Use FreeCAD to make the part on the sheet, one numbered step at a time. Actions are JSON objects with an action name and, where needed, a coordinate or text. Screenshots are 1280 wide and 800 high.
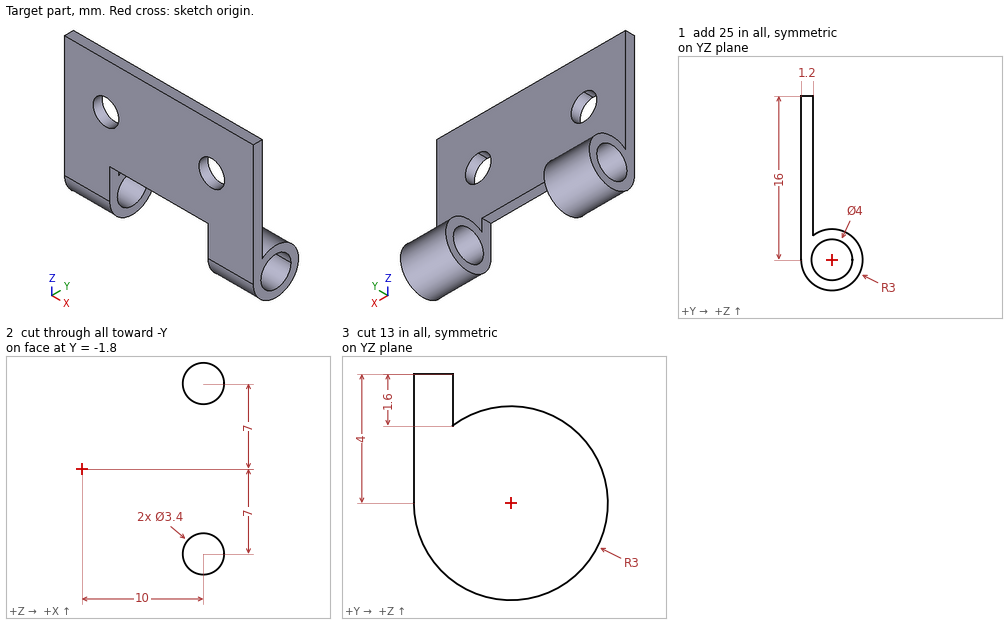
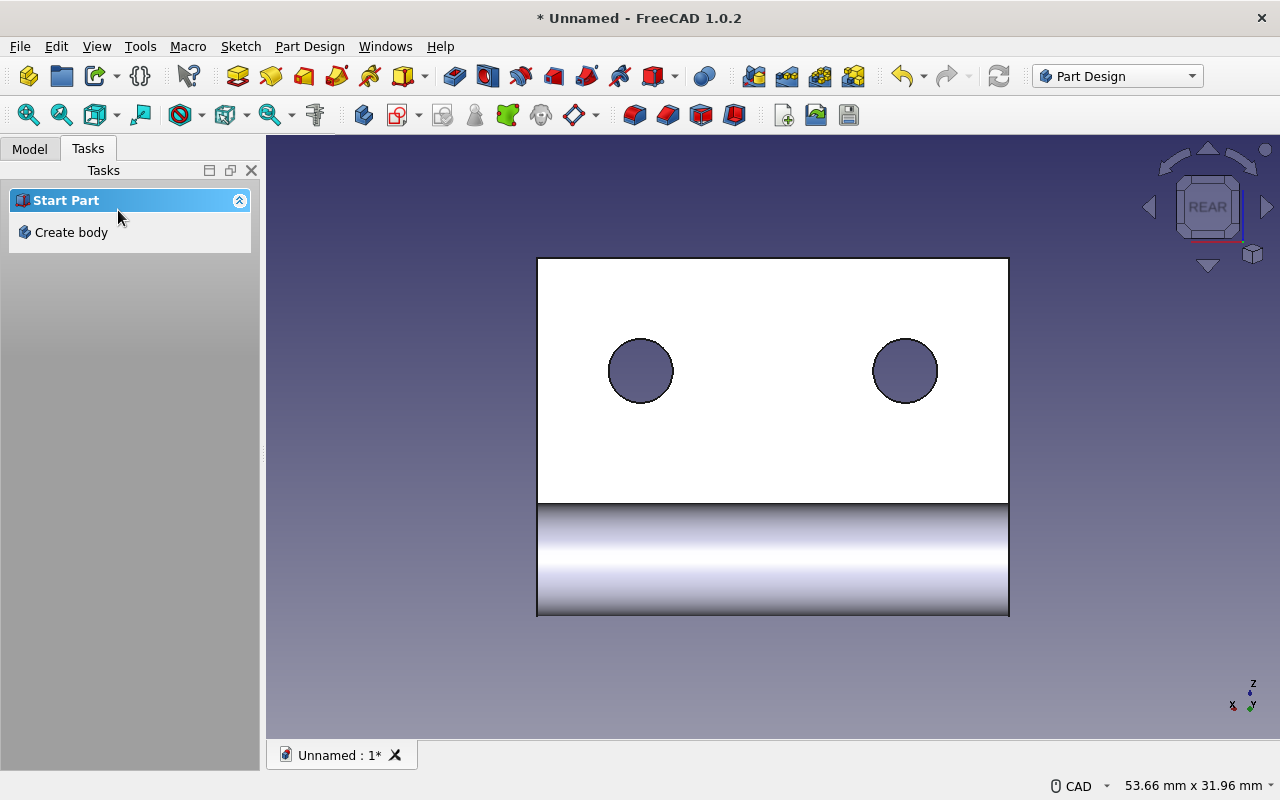
{"action": "left_click", "coordinate": [396, 116]}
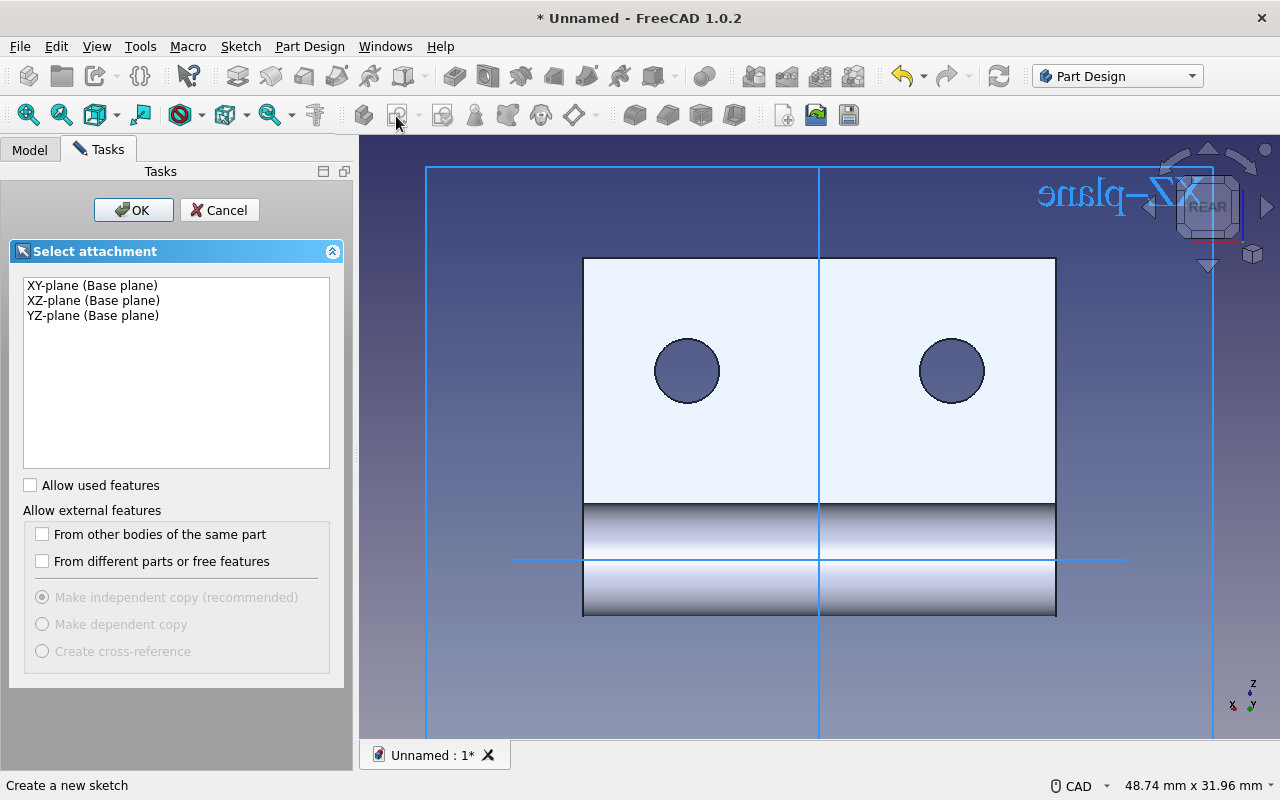
{"action": "left_click", "coordinate": [84, 316]}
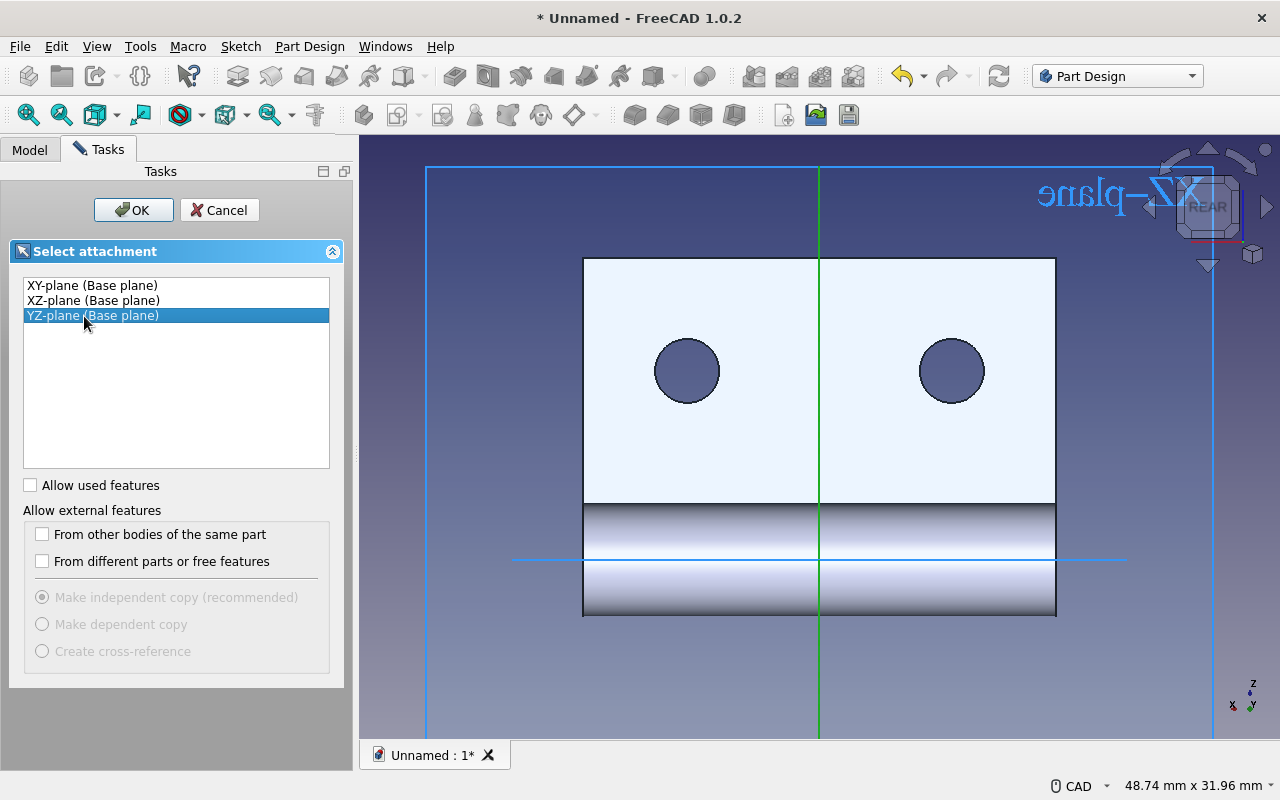
{"action": "left_click", "coordinate": [134, 210]}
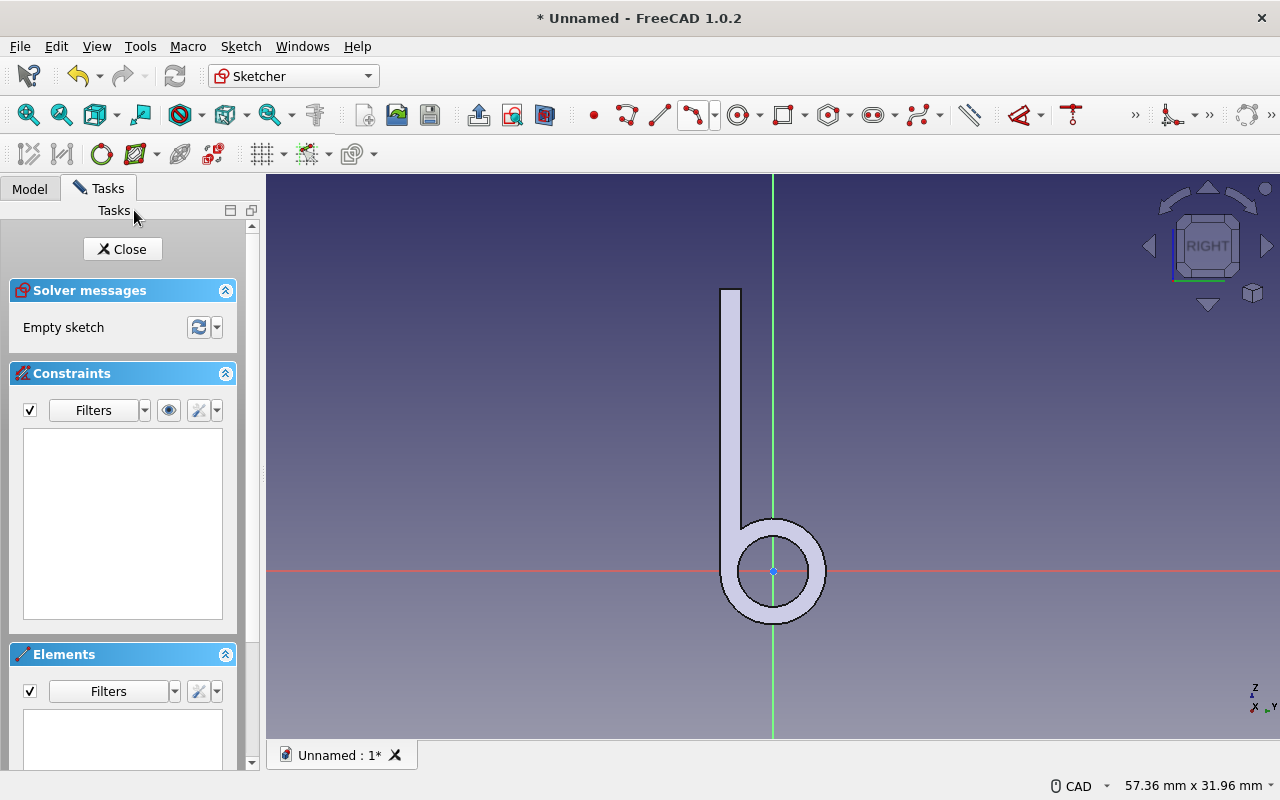
{"action": "left_click", "coordinate": [545, 116]}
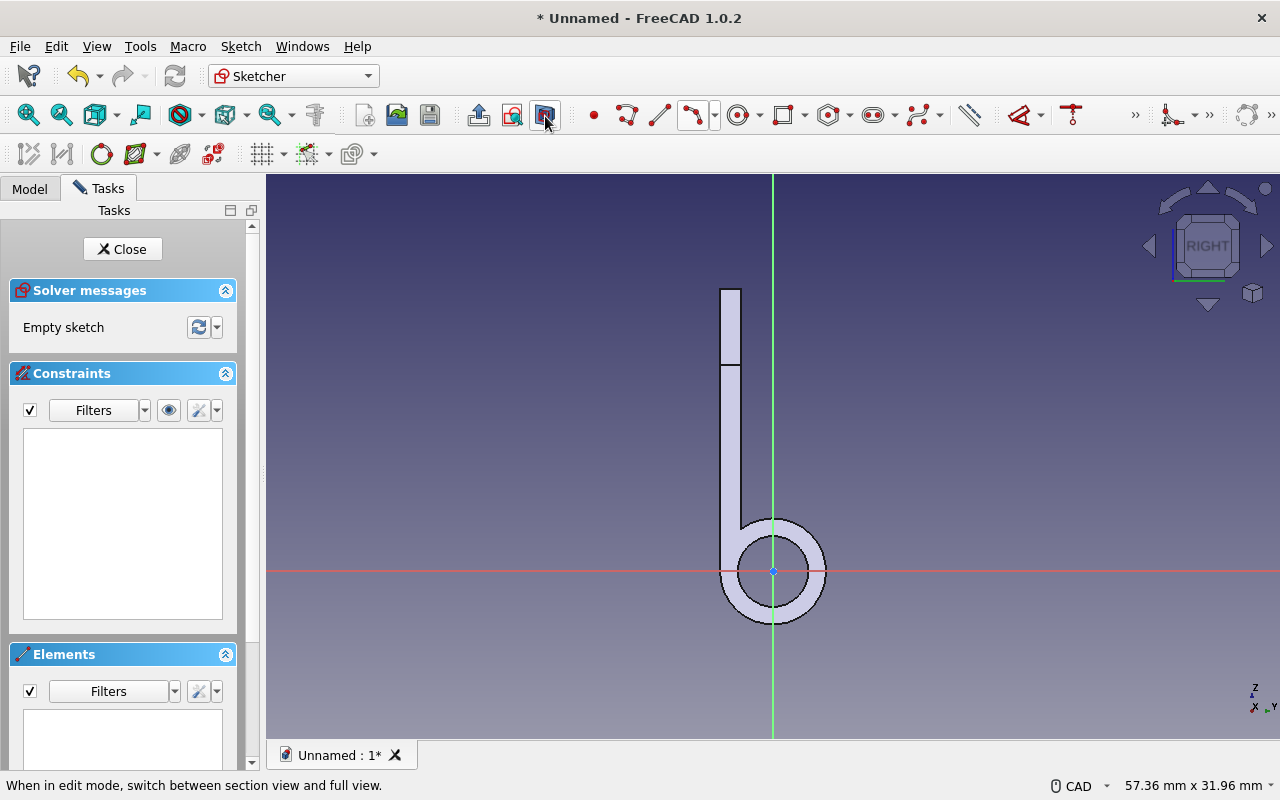
{"action": "scroll", "coordinate": [792, 578], "scroll_direction": "up", "scroll_amount": 7}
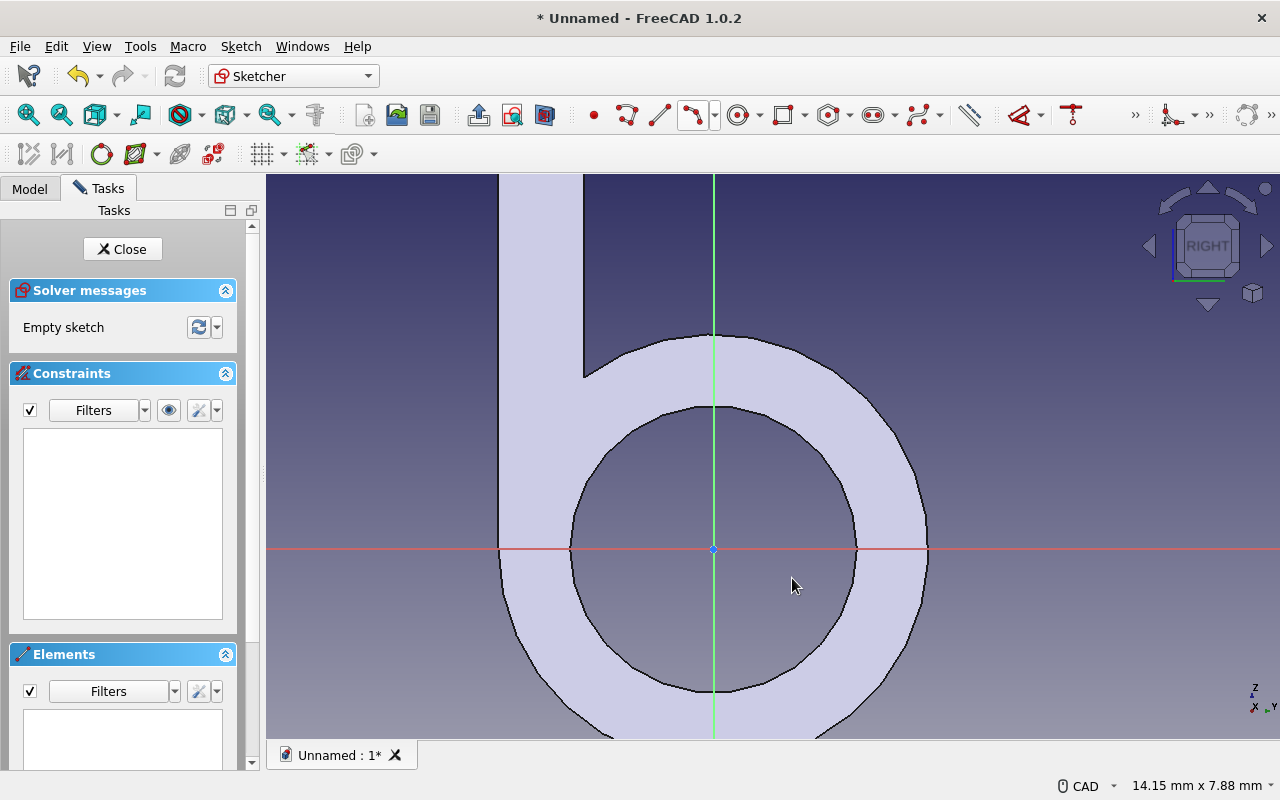
{"action": "left_click", "coordinate": [627, 116]}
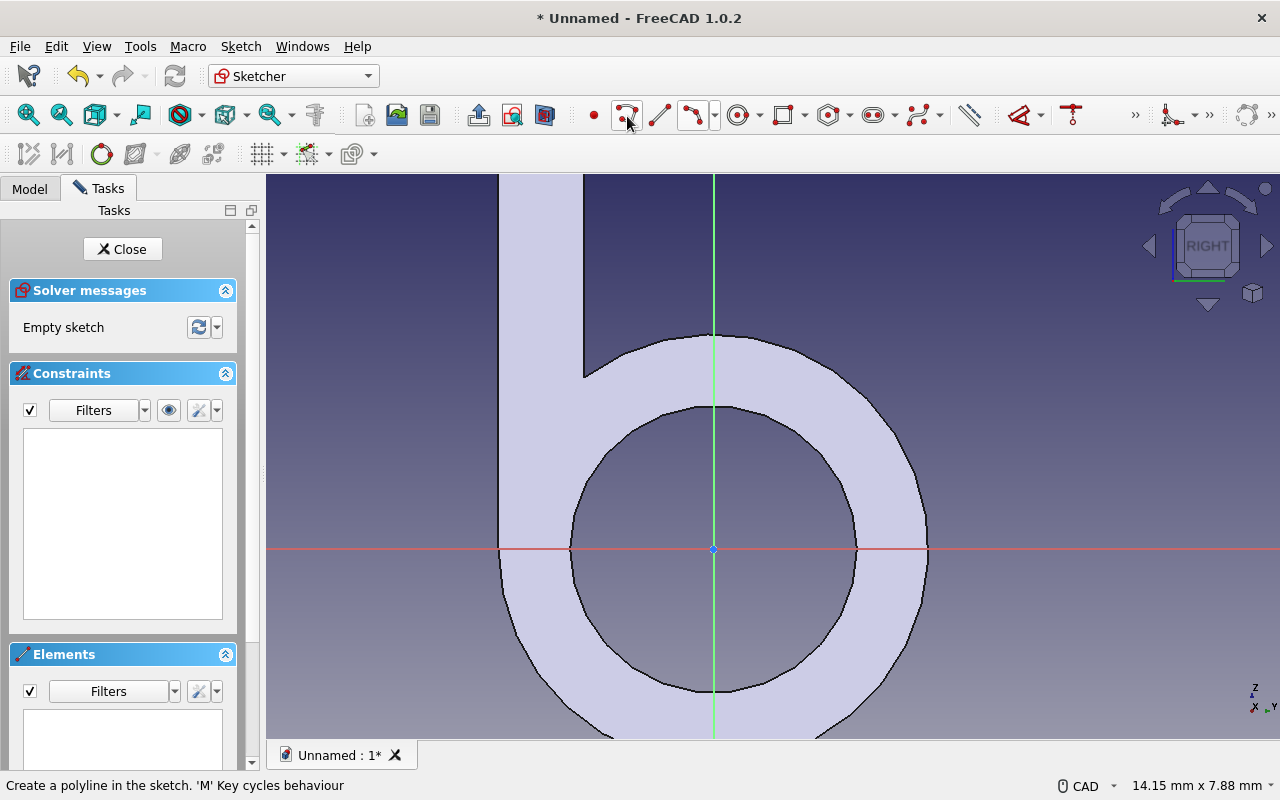
{"action": "left_click", "coordinate": [584, 377]}
{"action": "left_click", "coordinate": [584, 263]}
{"action": "left_click", "coordinate": [498, 263]}
{"action": "left_click", "coordinate": [498, 549]}
{"action": "right_click", "coordinate": [498, 549]}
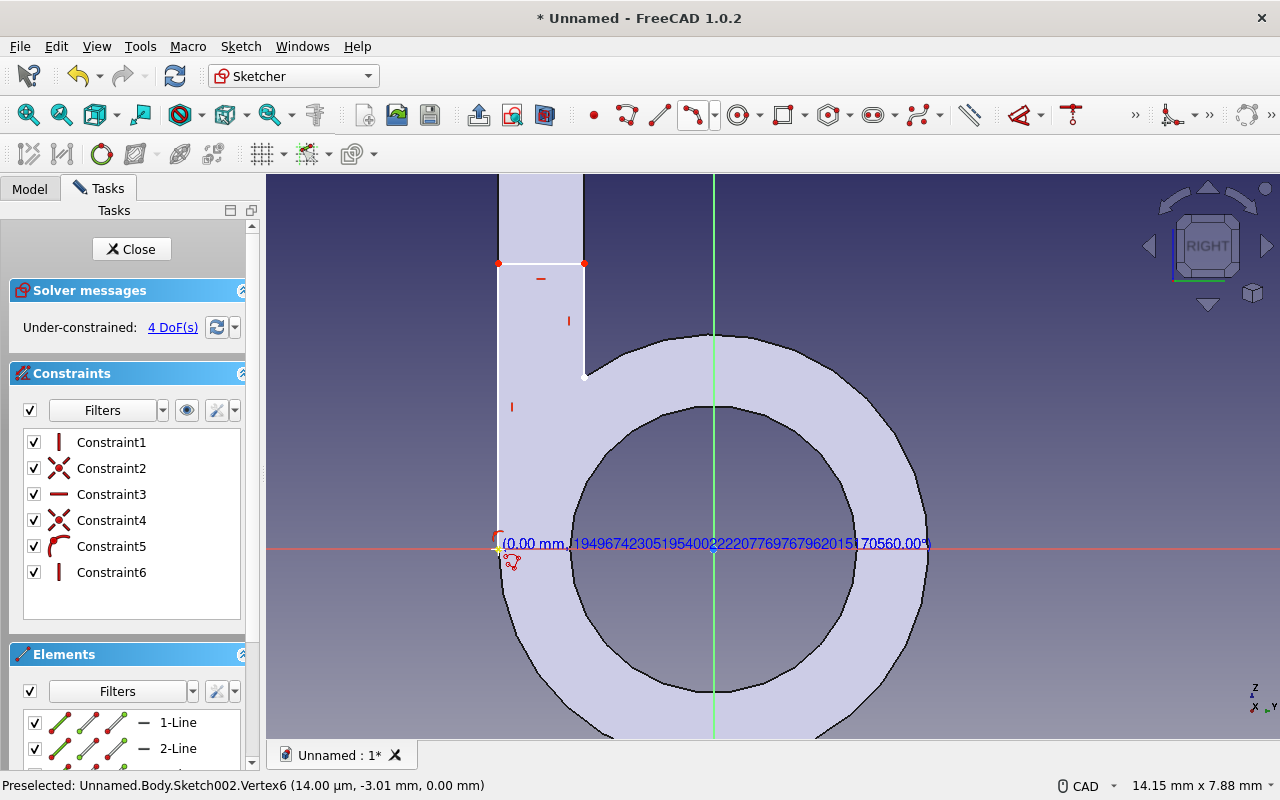
{"action": "left_click", "coordinate": [692, 116]}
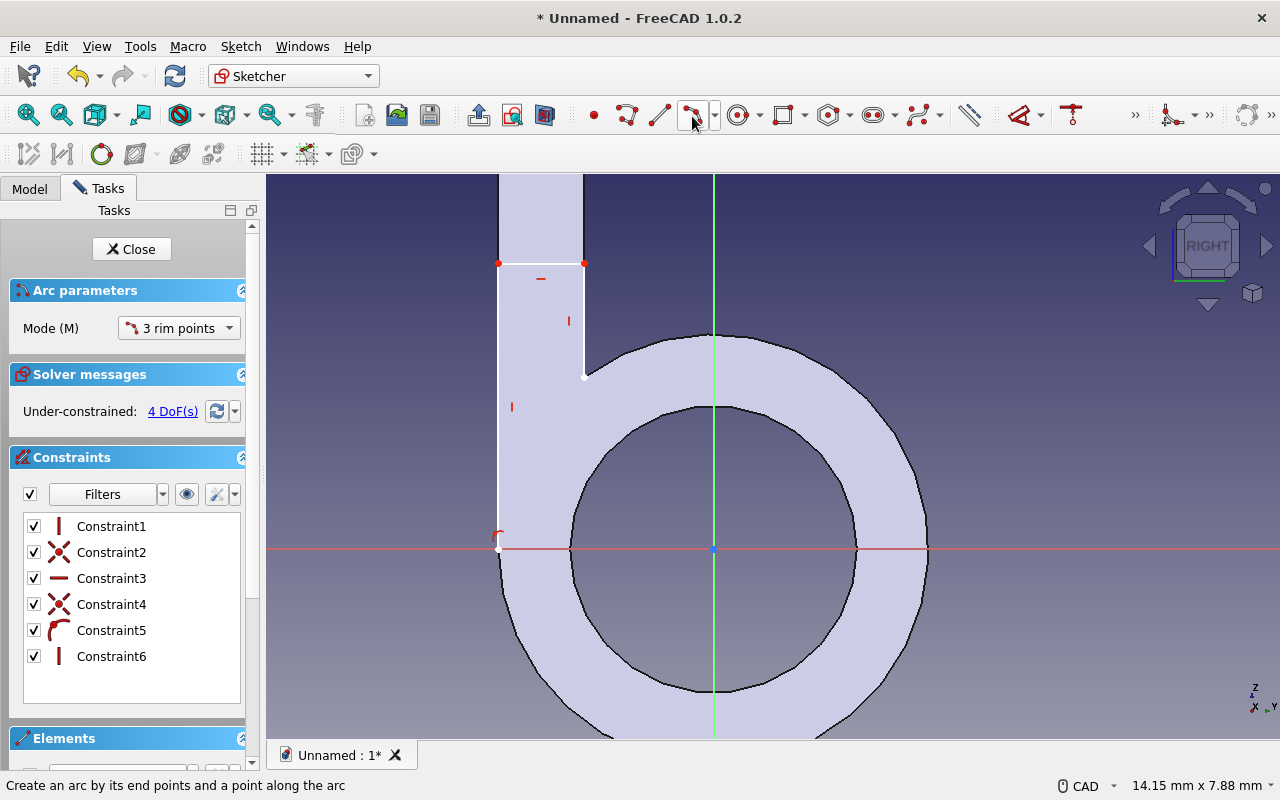
{"action": "left_click", "coordinate": [498, 549]}
{"action": "left_click", "coordinate": [584, 378]}
{"action": "left_click", "coordinate": [906, 646]}
{"action": "key", "text": "Escape"}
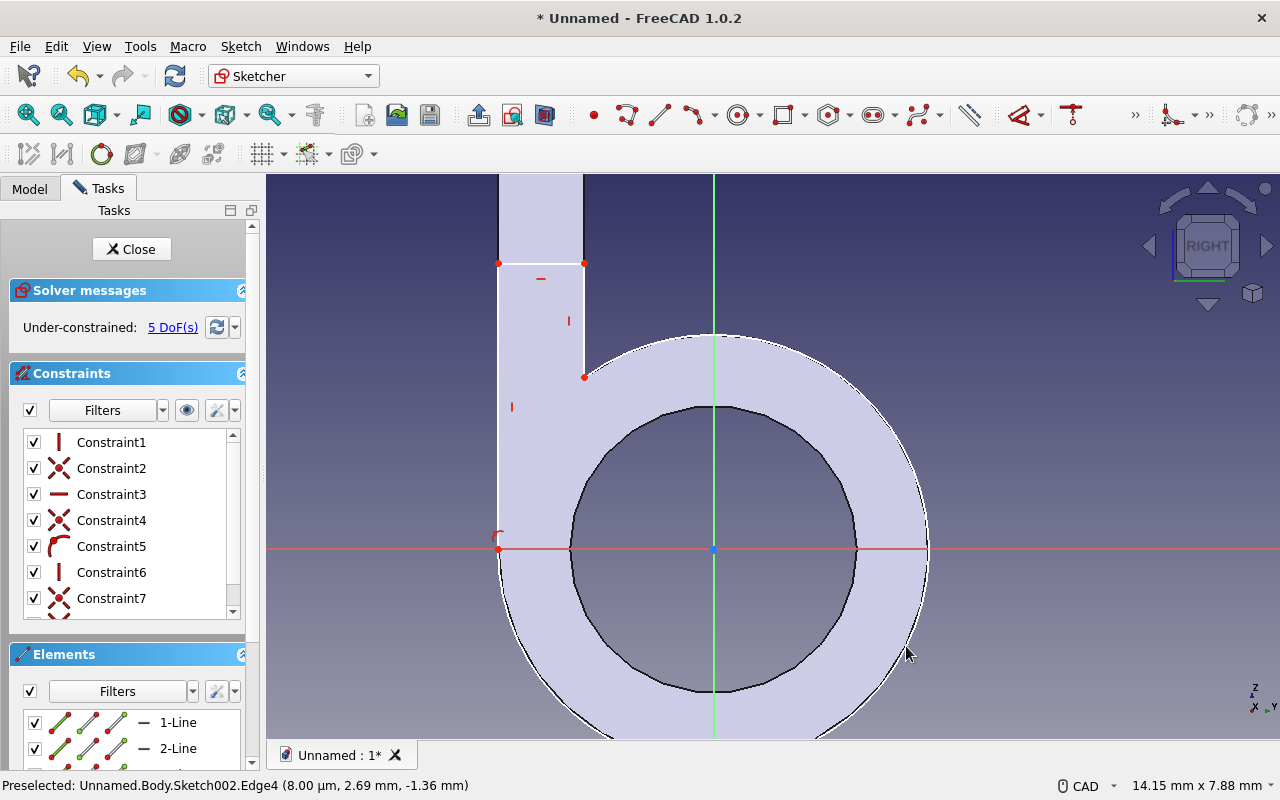
{"action": "left_click", "coordinate": [498, 350]}